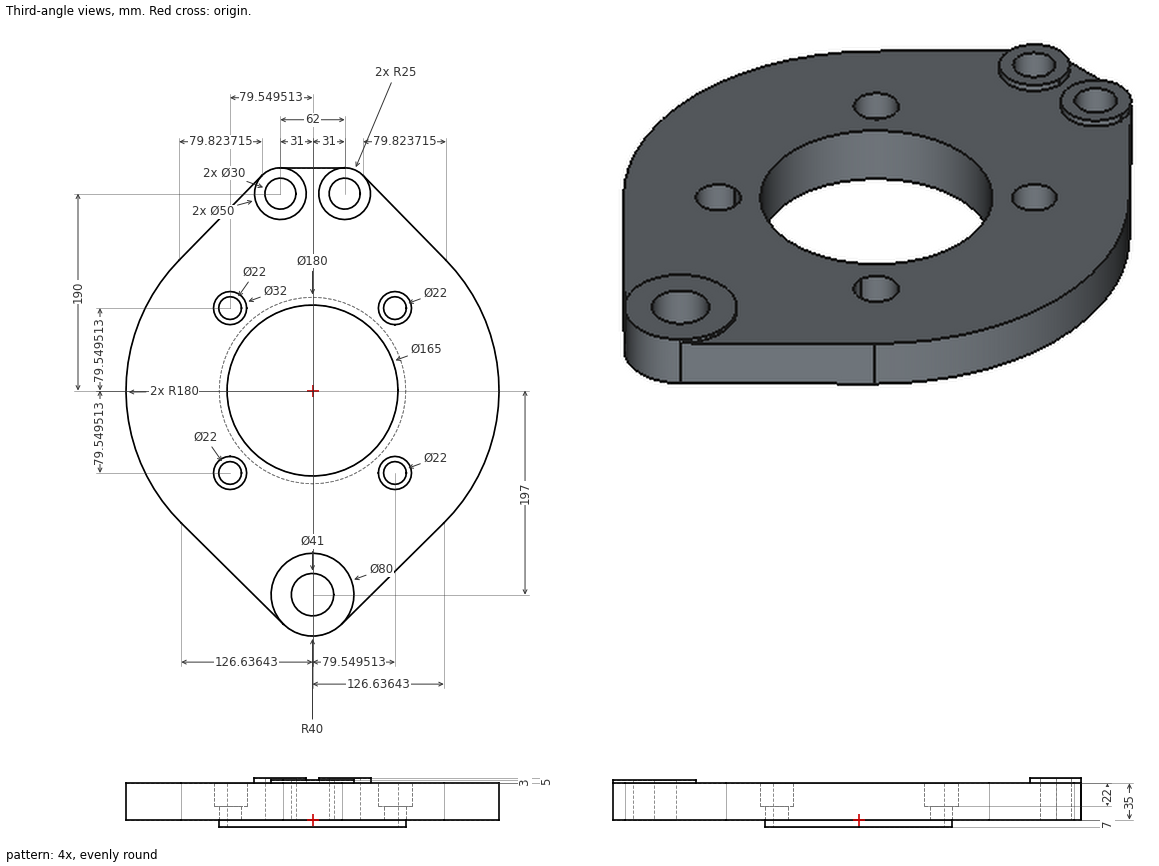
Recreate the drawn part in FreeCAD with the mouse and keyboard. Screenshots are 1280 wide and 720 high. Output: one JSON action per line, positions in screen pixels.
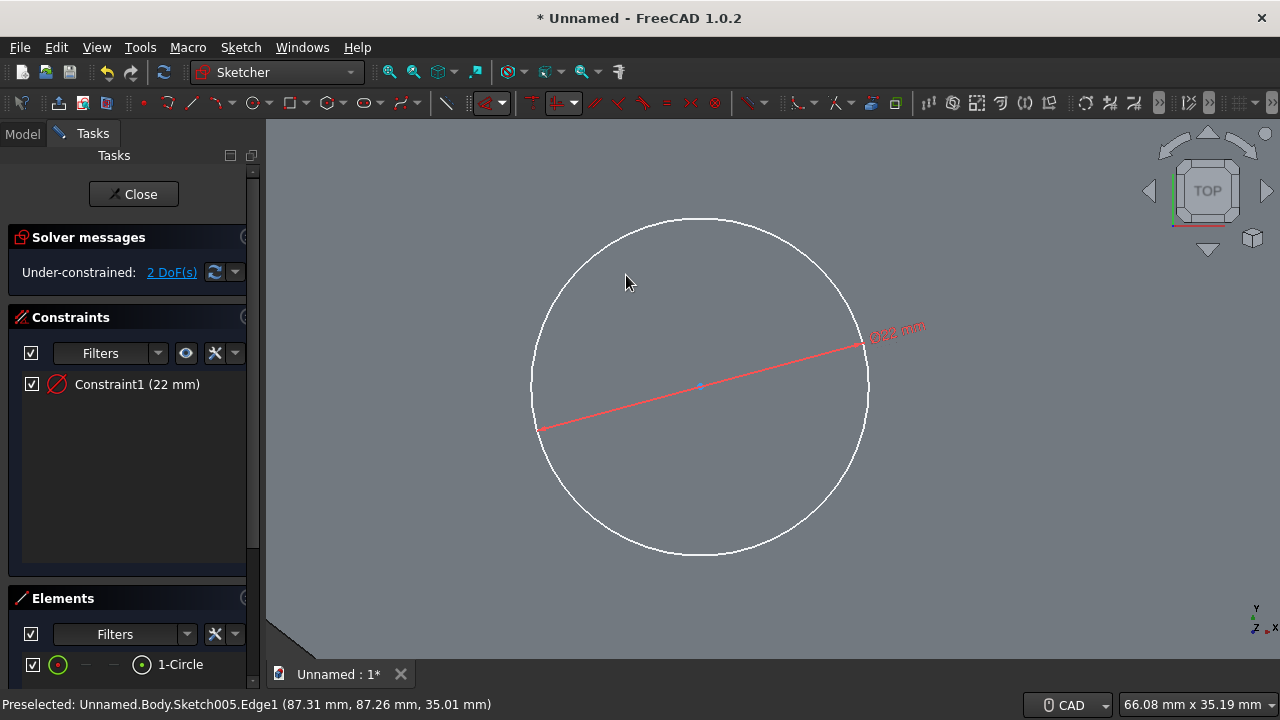
{"action": "left_click", "coordinate": [700, 387]}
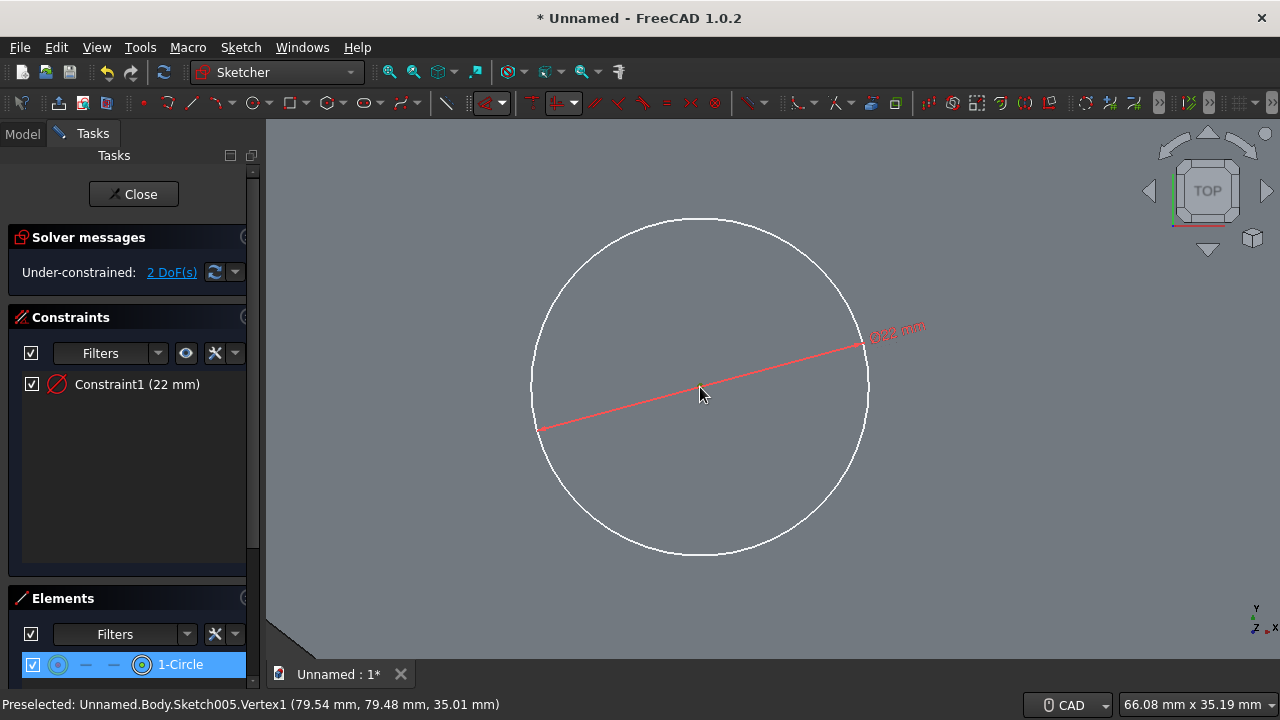
{"action": "key", "text": "l"}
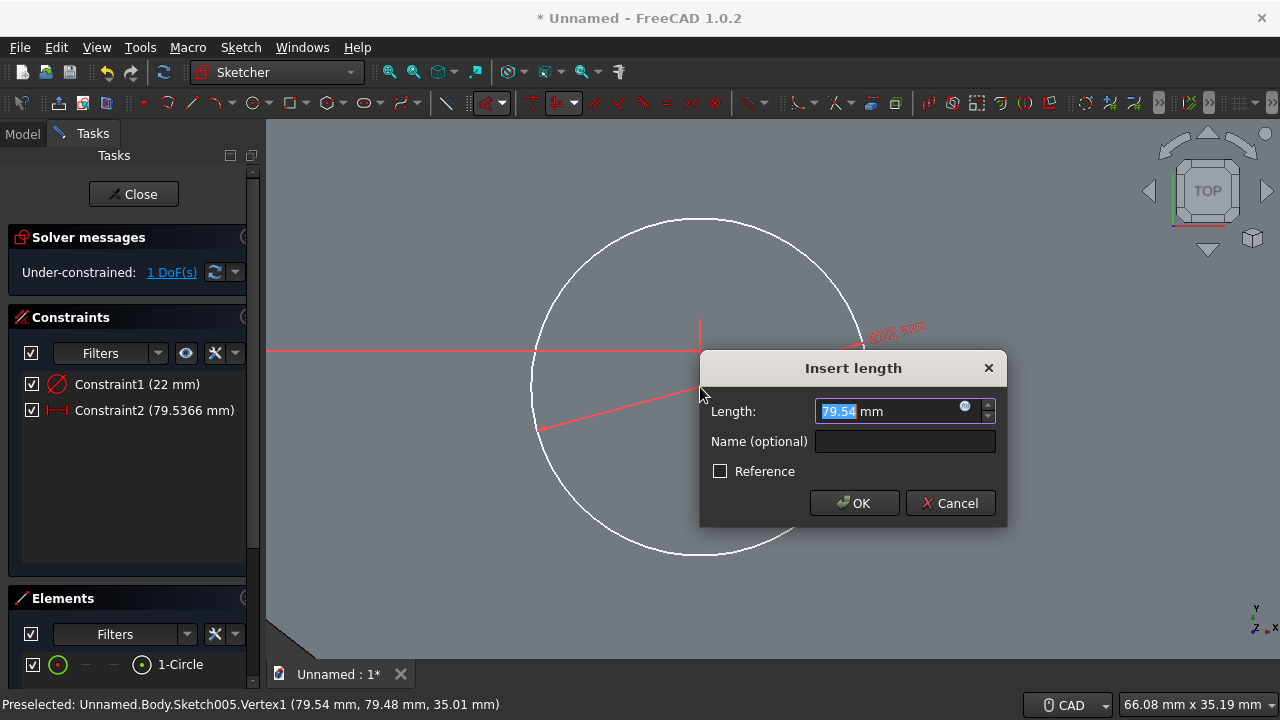
{"action": "type", "text": "79.549513"}
{"action": "key", "text": "Return"}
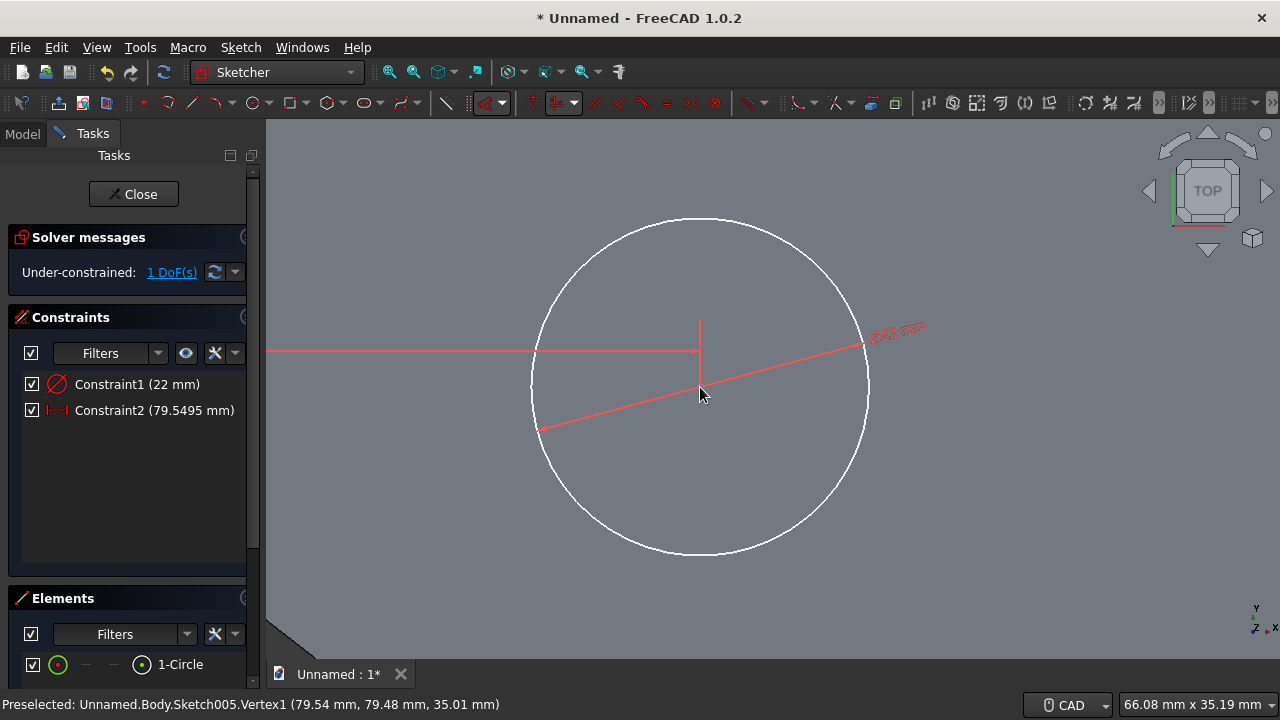
{"action": "left_click", "coordinate": [700, 387]}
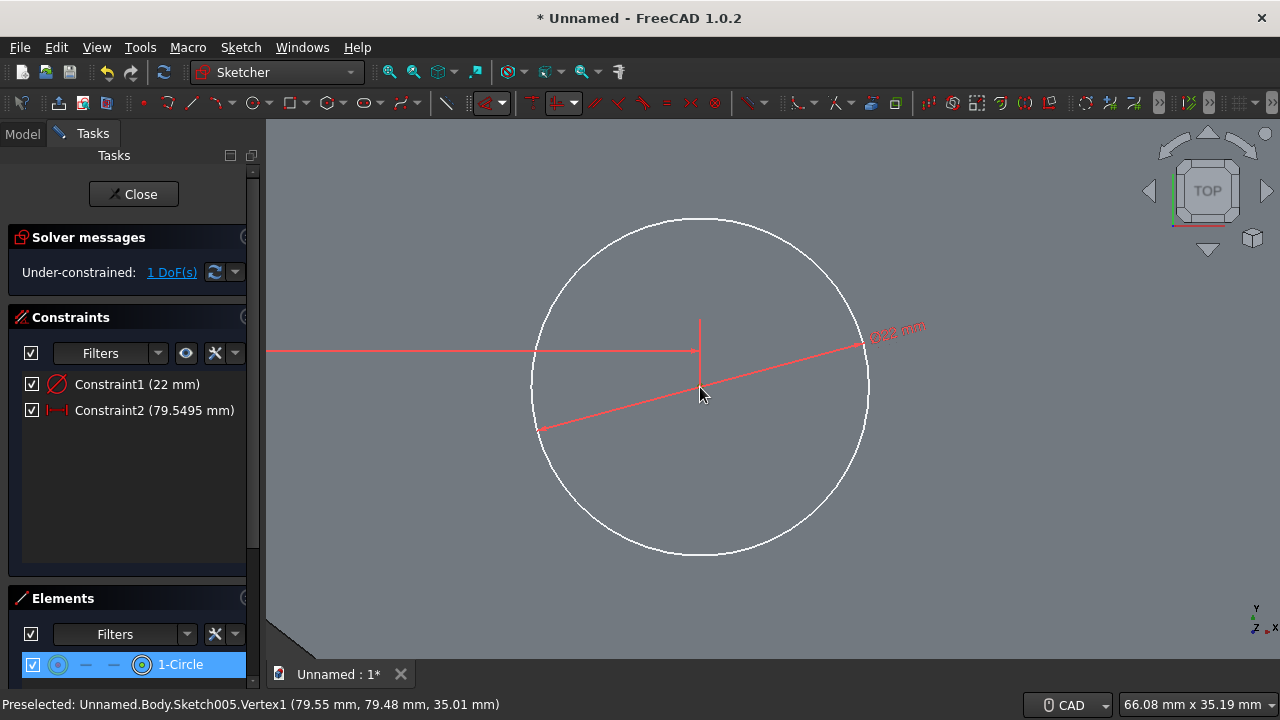
{"action": "key", "text": "i"}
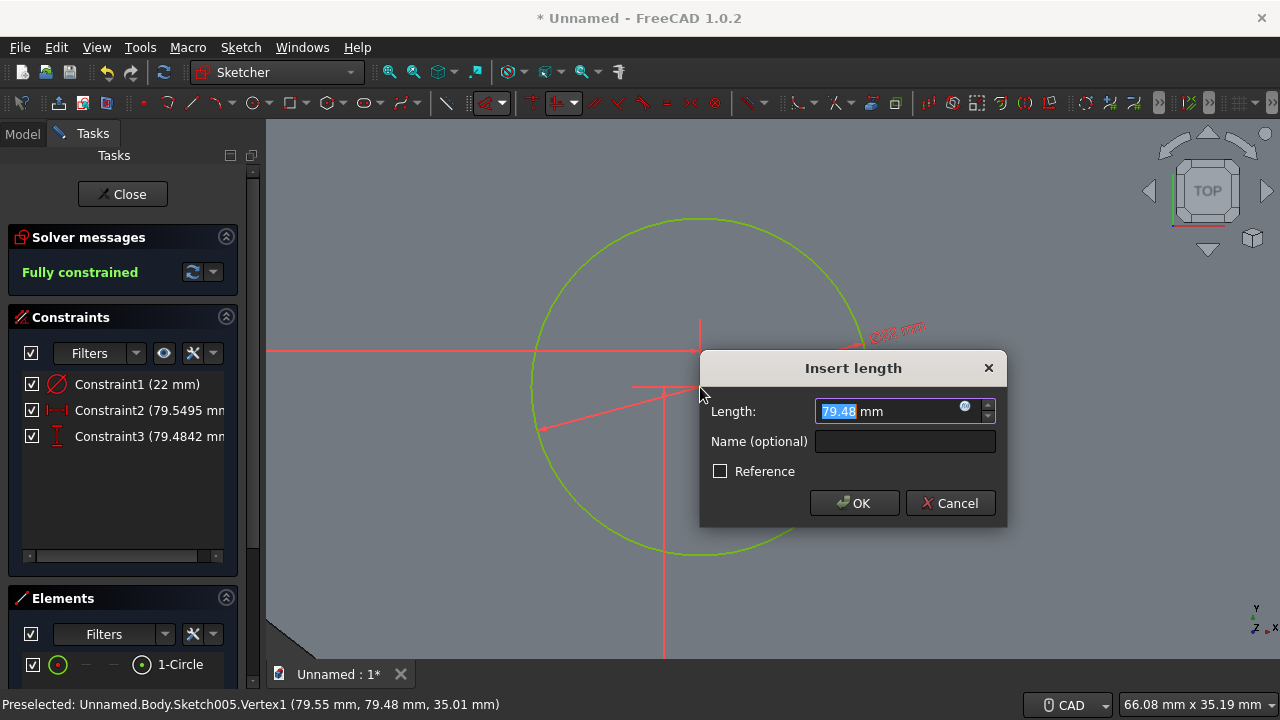
{"action": "type", "text": "79.549513"}
{"action": "key", "text": "Return"}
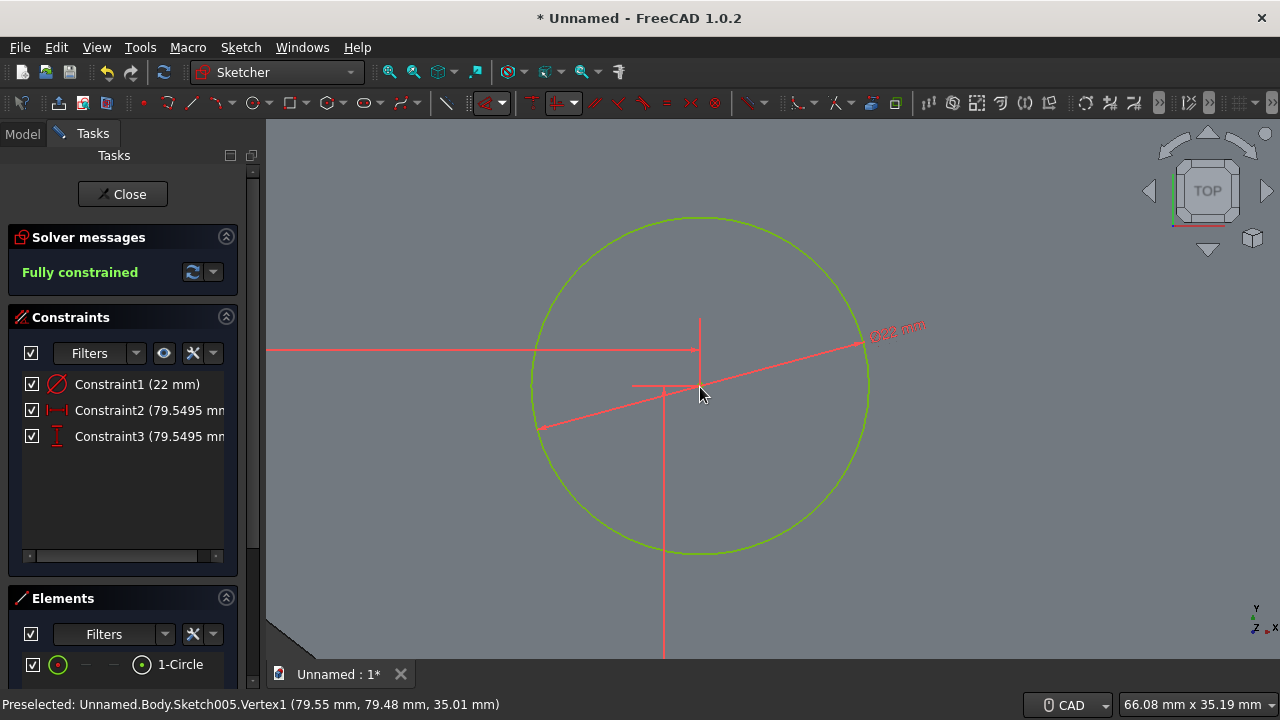
{"action": "left_click", "coordinate": [123, 194]}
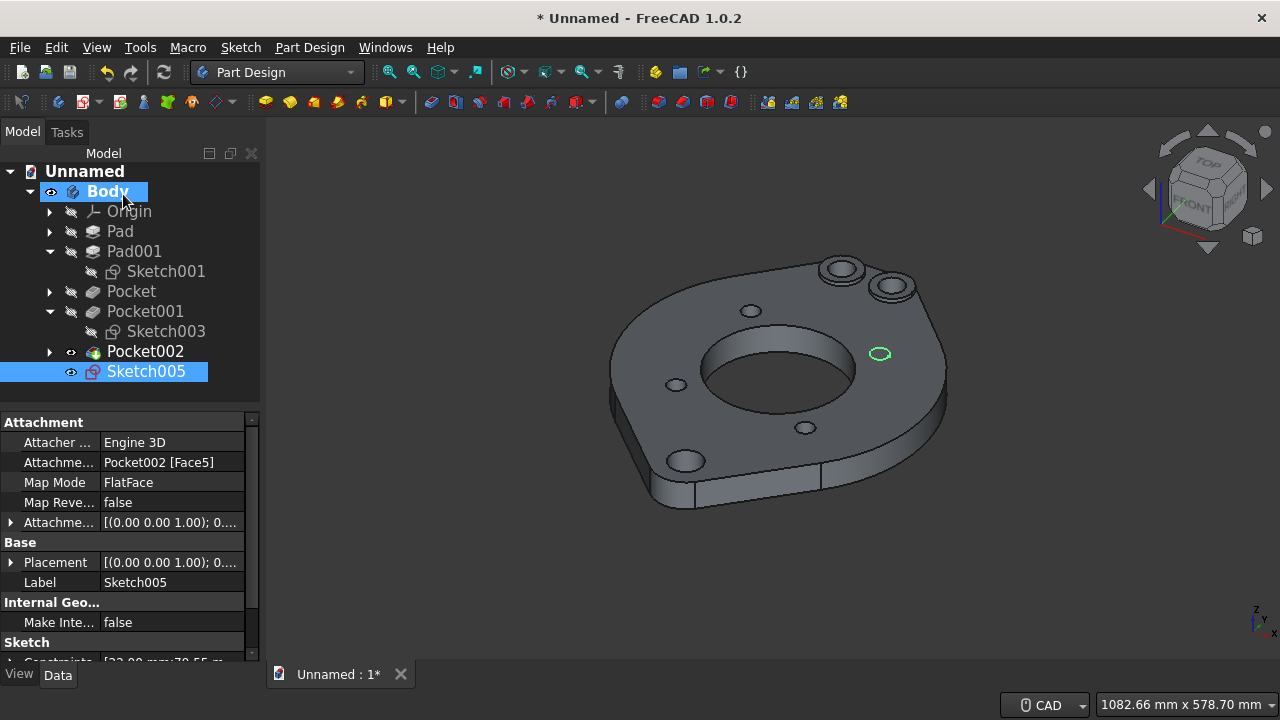
{"action": "left_click", "coordinate": [432, 102]}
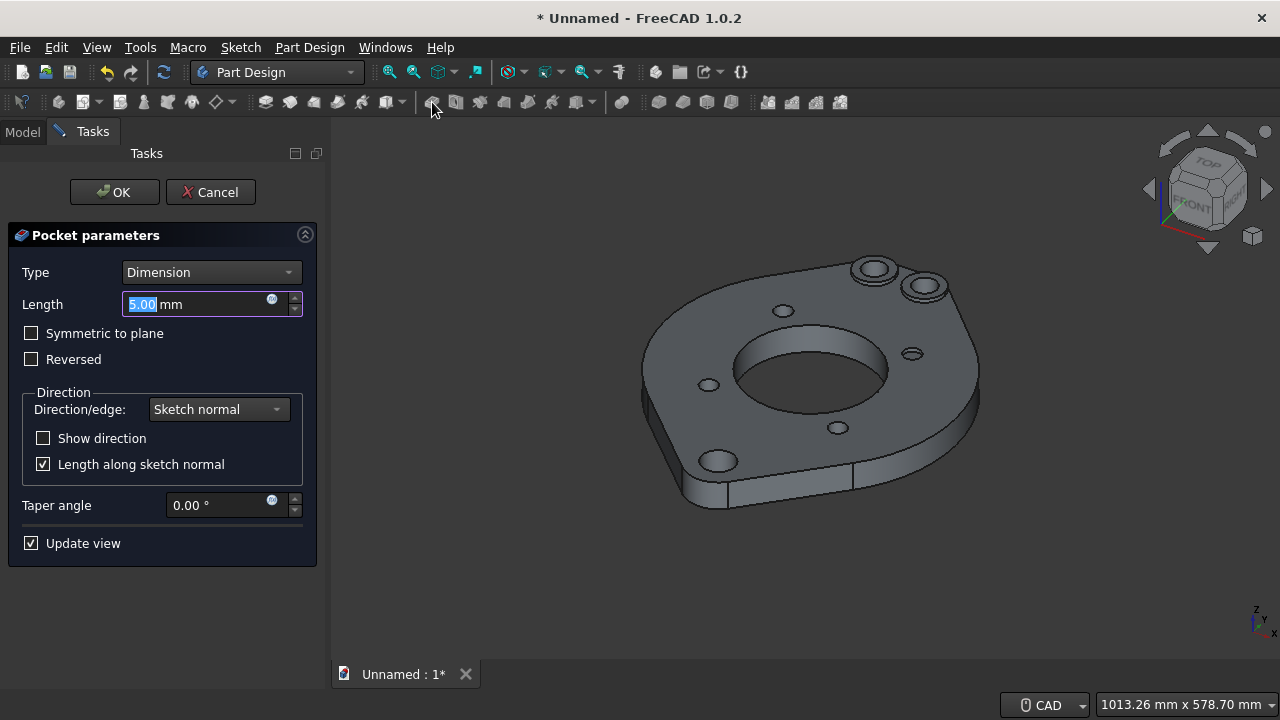
{"action": "left_click", "coordinate": [212, 272]}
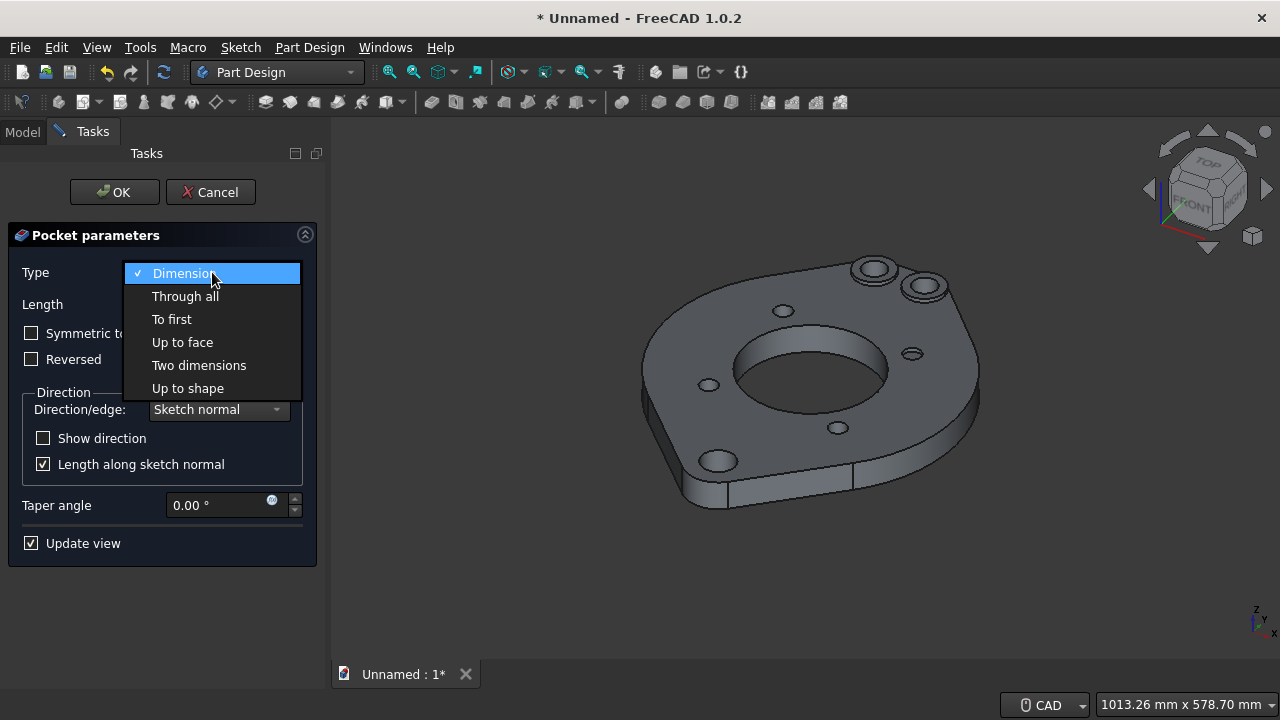
{"action": "left_click", "coordinate": [212, 320]}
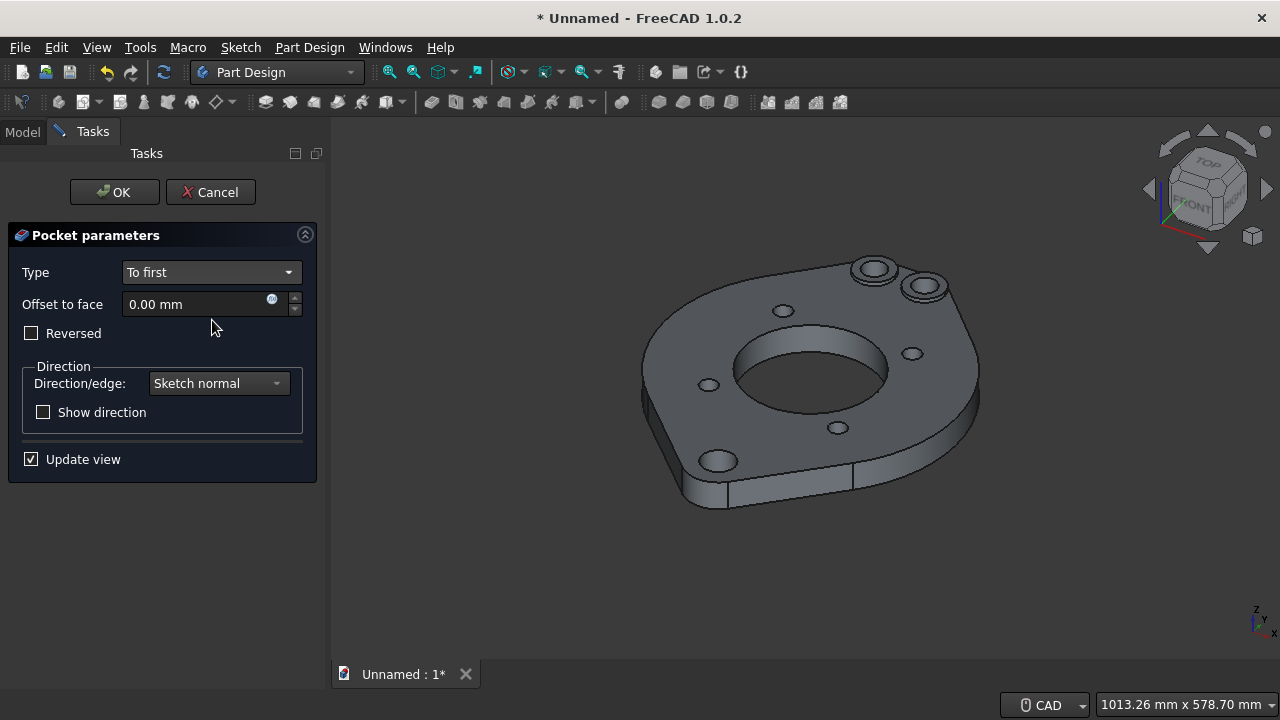
{"action": "left_click", "coordinate": [115, 192]}